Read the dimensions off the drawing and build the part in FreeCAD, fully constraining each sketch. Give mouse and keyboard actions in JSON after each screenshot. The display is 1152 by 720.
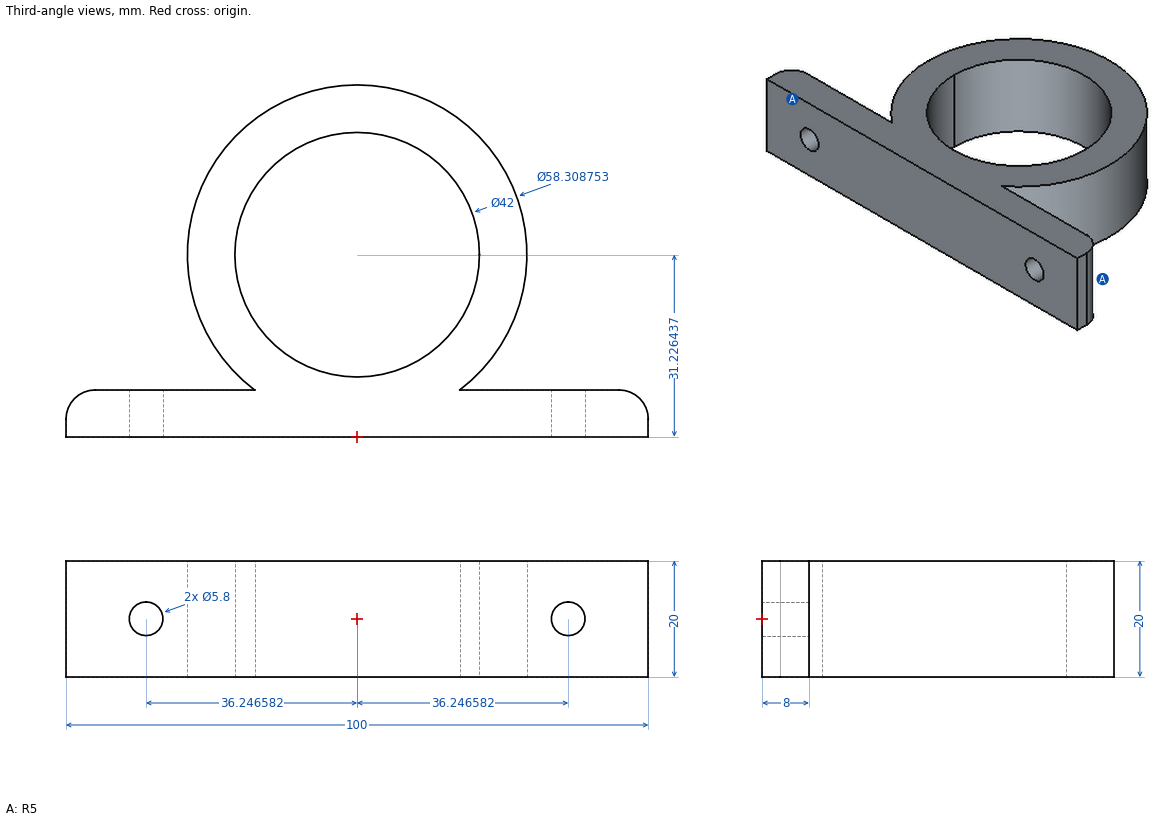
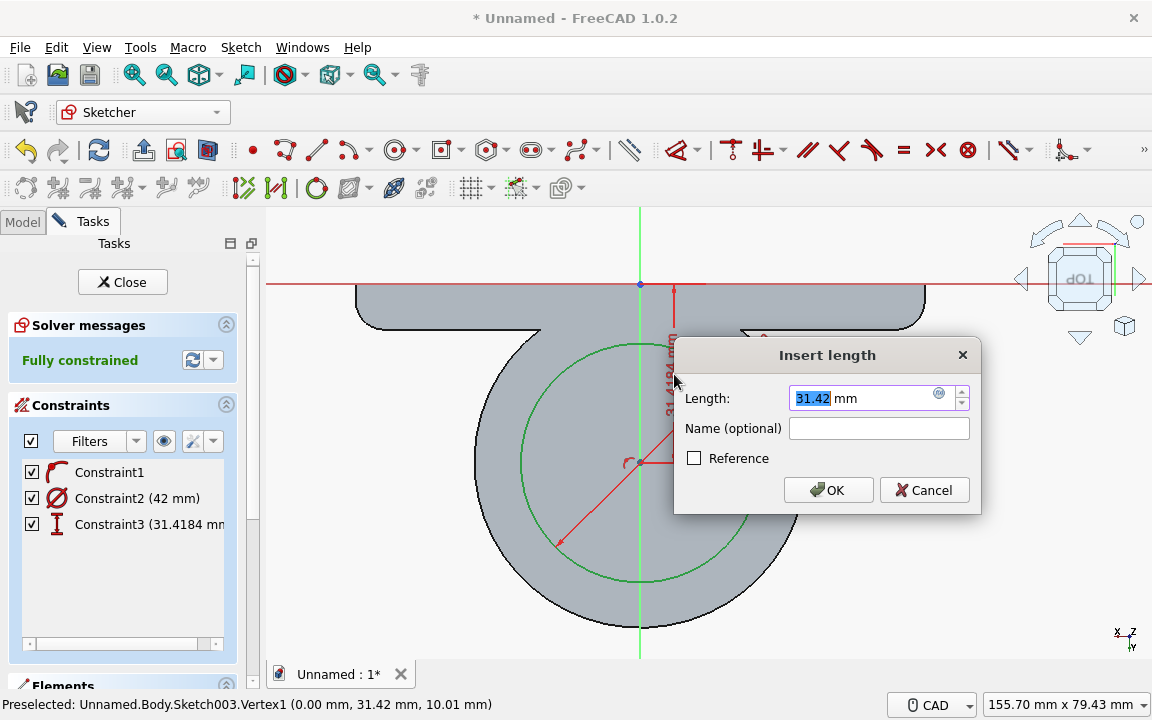
{"action": "type", "text": "31.226437"}
{"action": "key", "text": "Return"}
{"action": "key", "text": "Escape"}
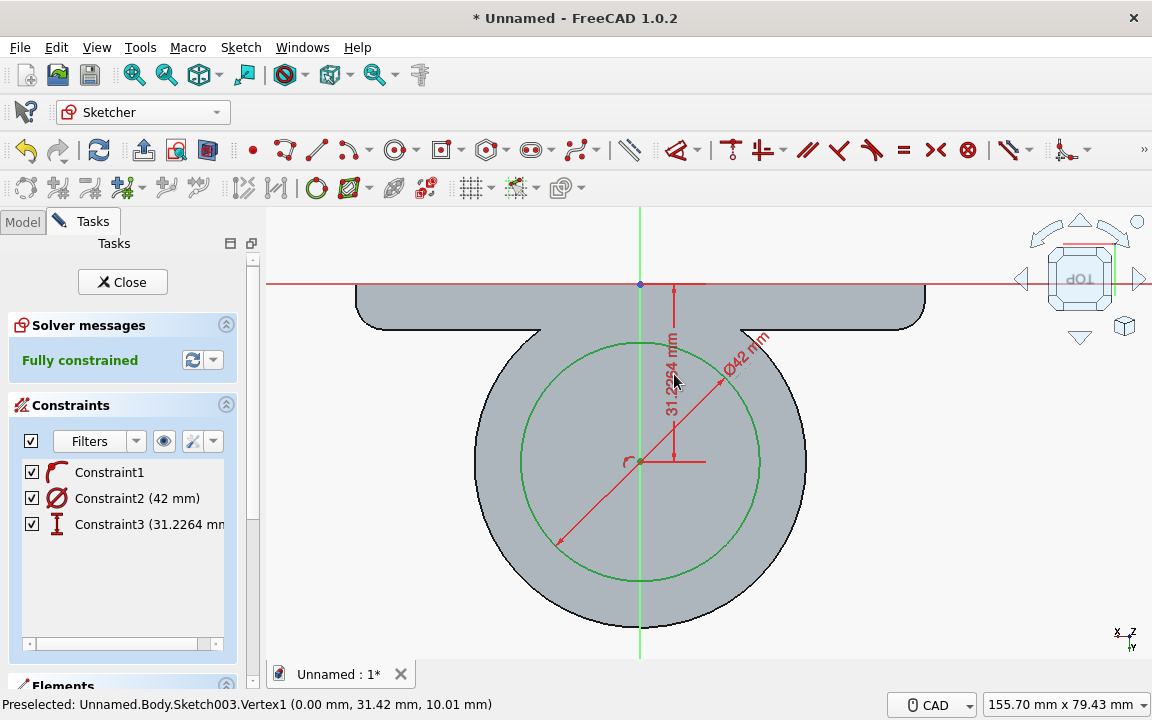
{"action": "left_click", "coordinate": [123, 282]}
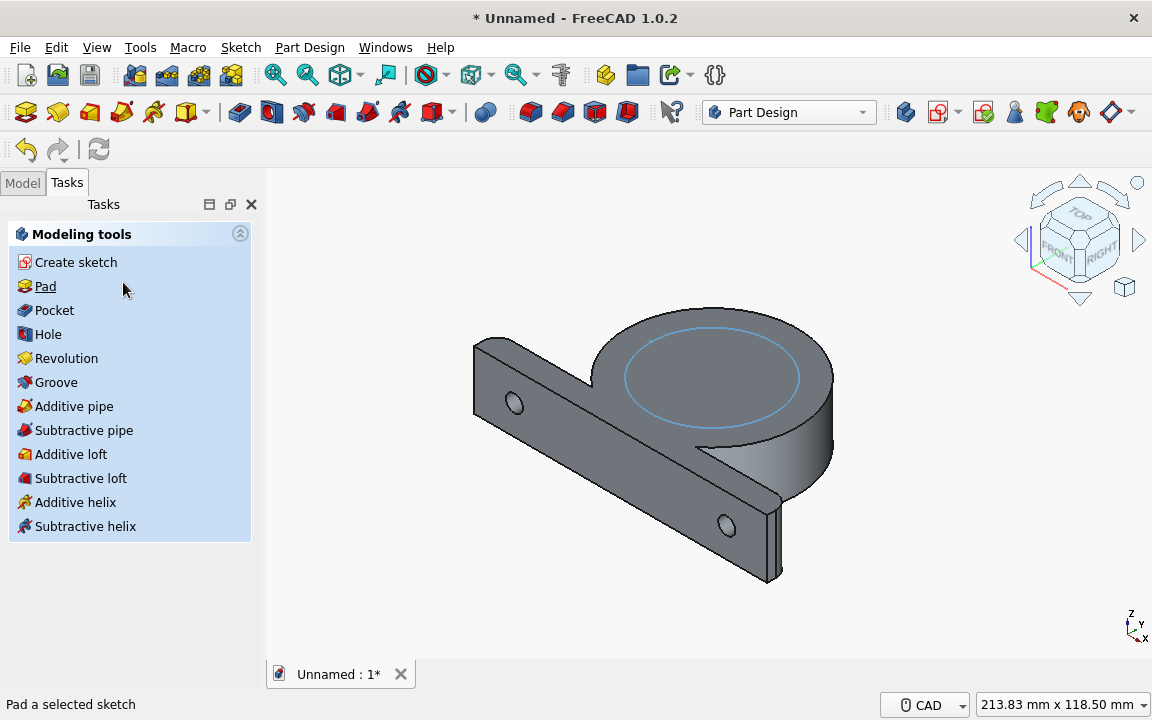
{"action": "left_click", "coordinate": [240, 112]}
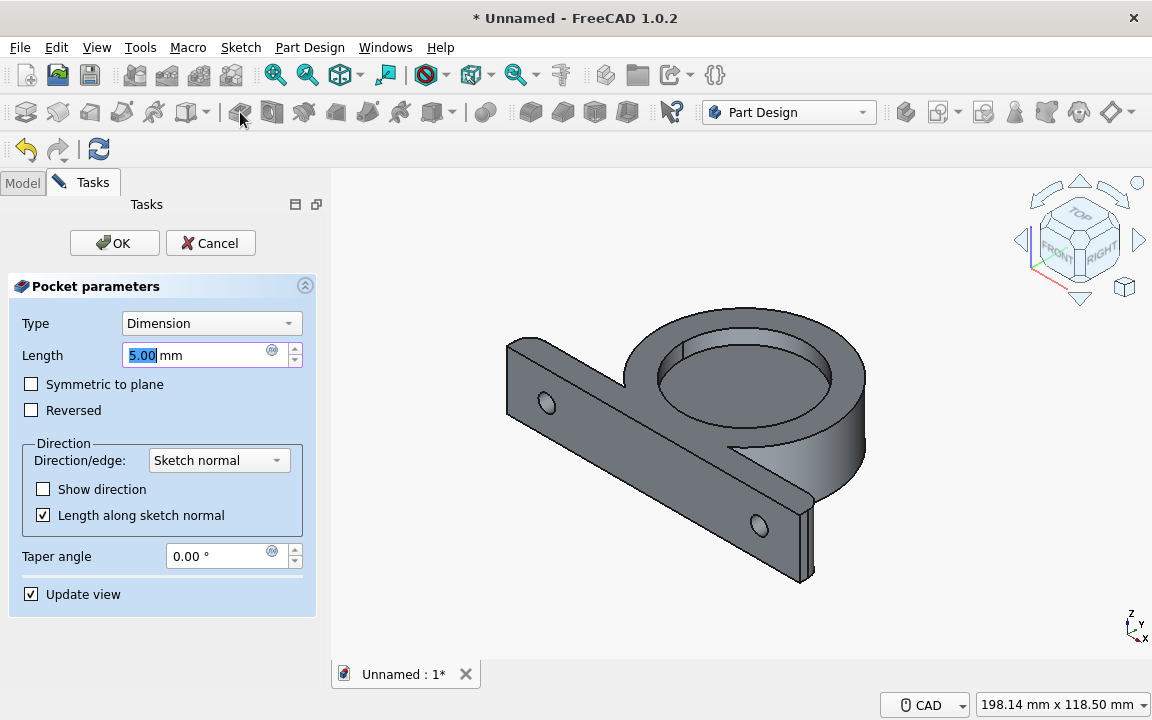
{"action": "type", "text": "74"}
{"action": "key", "text": "Tab"}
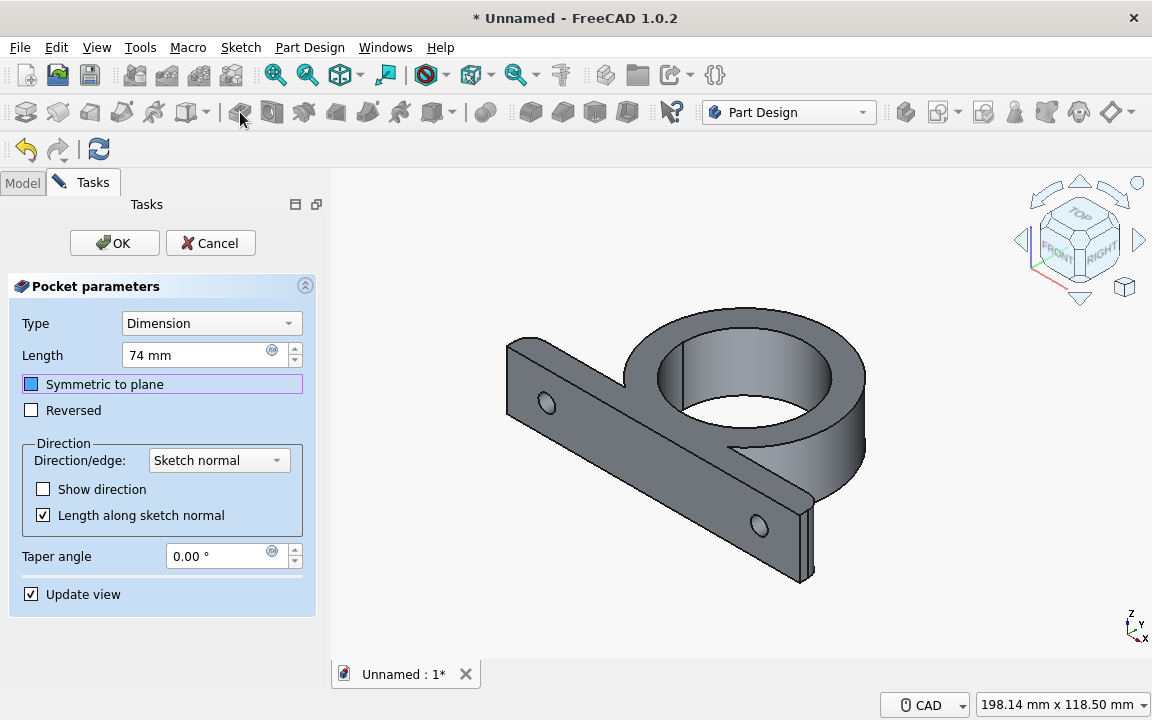
{"action": "left_click", "coordinate": [115, 243]}